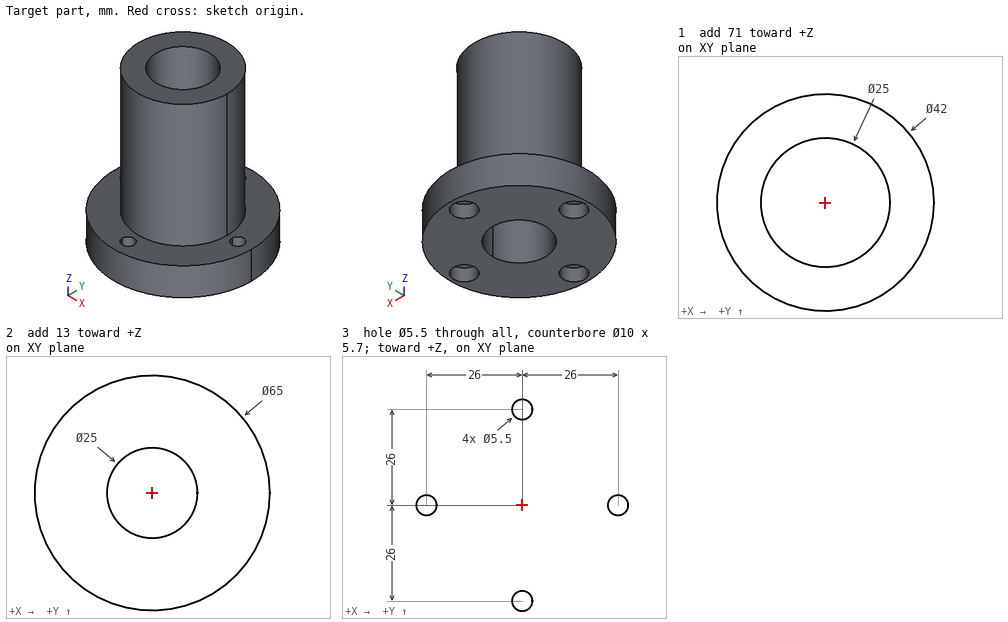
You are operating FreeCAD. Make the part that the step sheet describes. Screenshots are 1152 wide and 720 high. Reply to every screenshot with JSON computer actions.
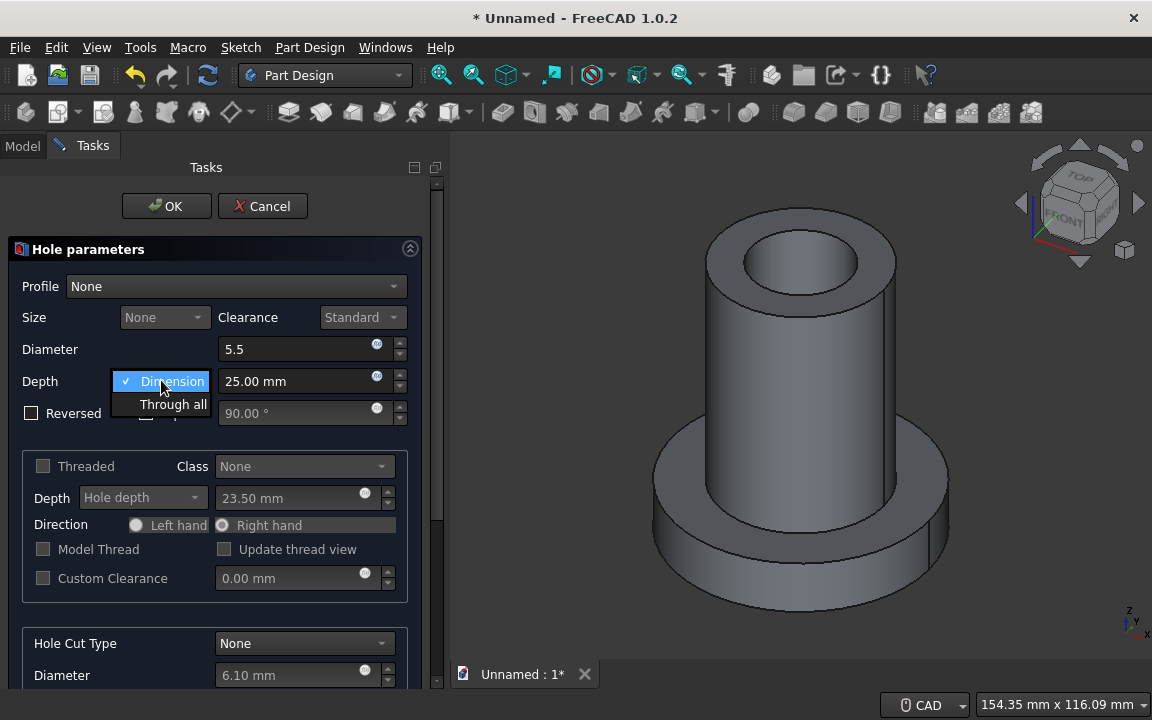
{"action": "left_click", "coordinate": [160, 404]}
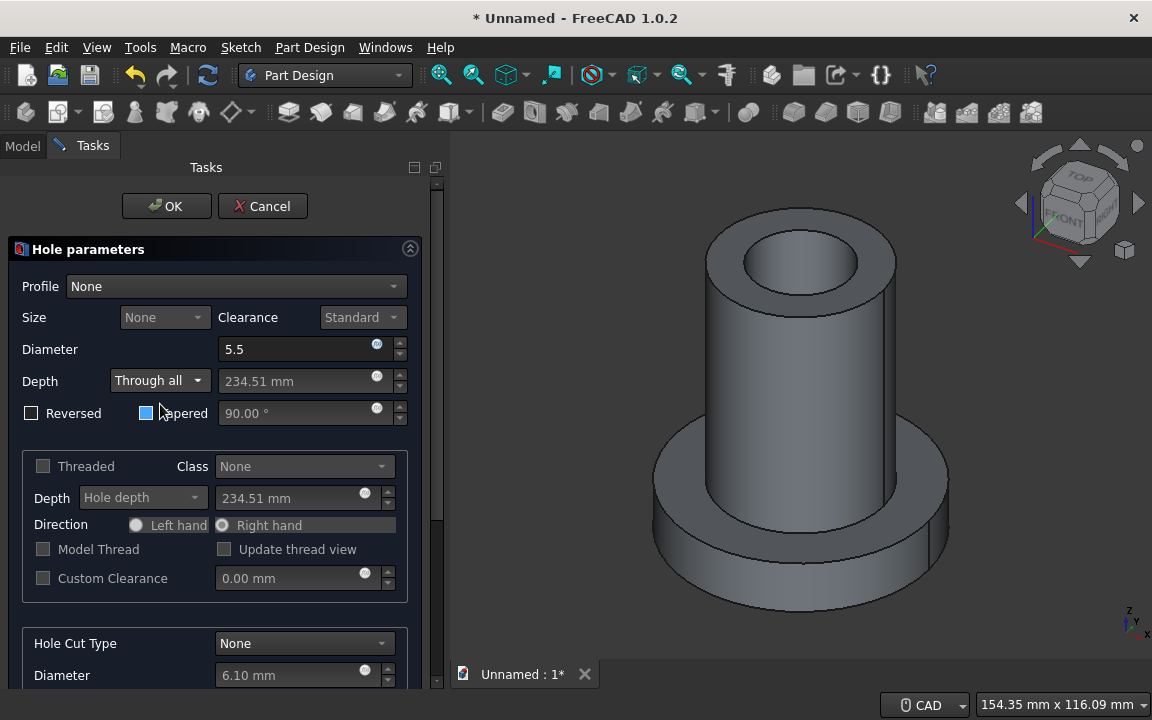
{"action": "left_click", "coordinate": [30, 413]}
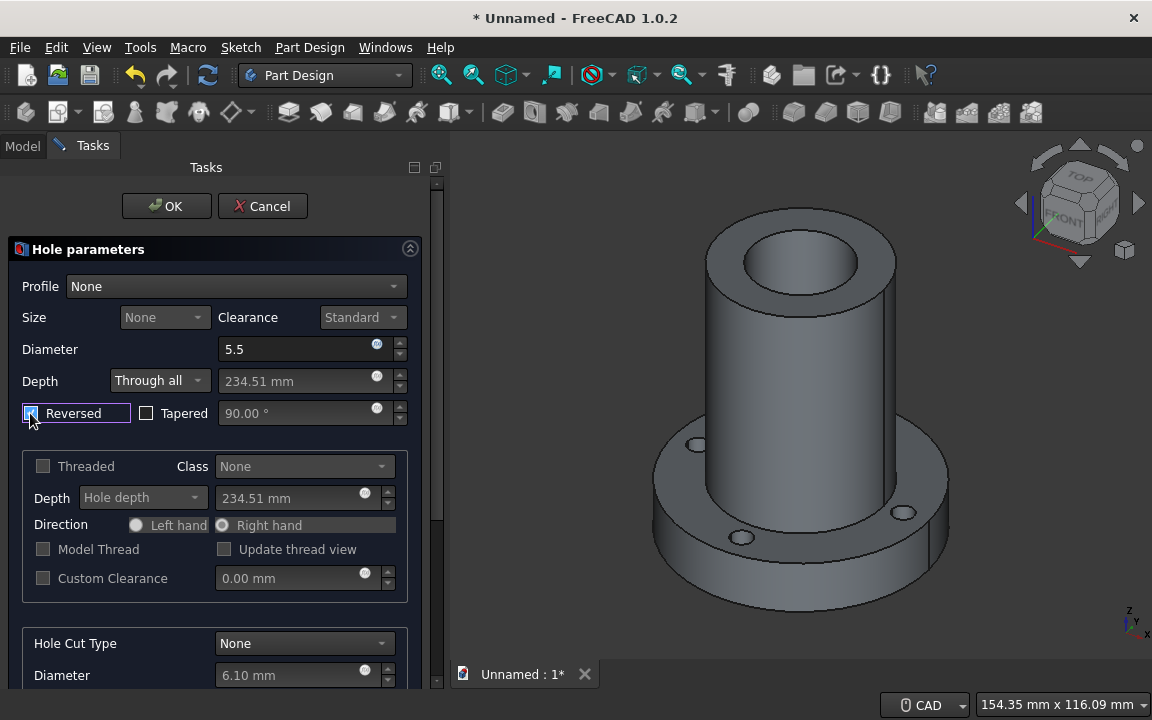
{"action": "left_click", "coordinate": [306, 644]}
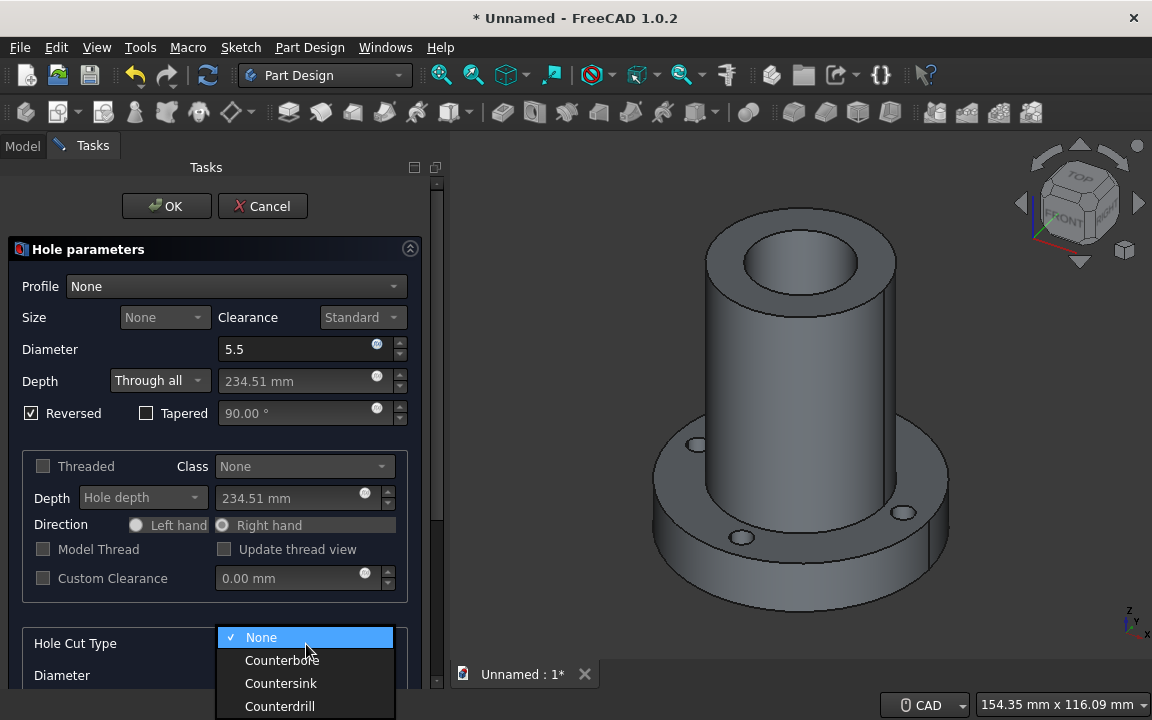
{"action": "left_click", "coordinate": [304, 660]}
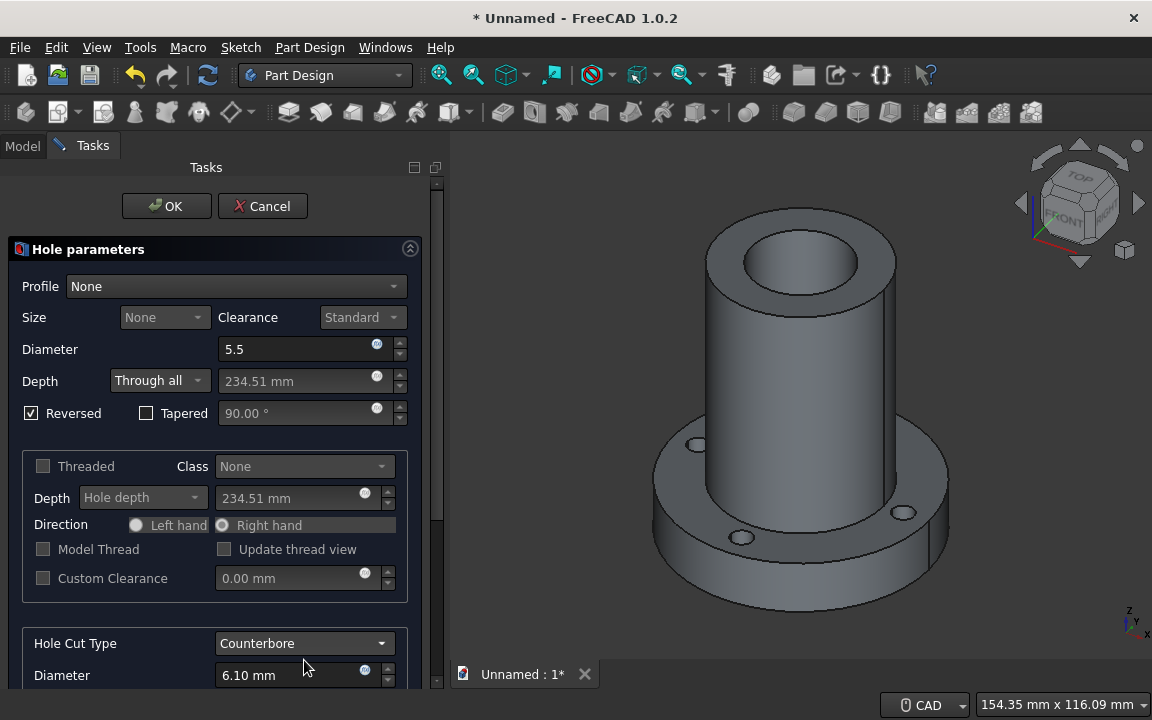
{"action": "triple_click", "coordinate": [298, 675]}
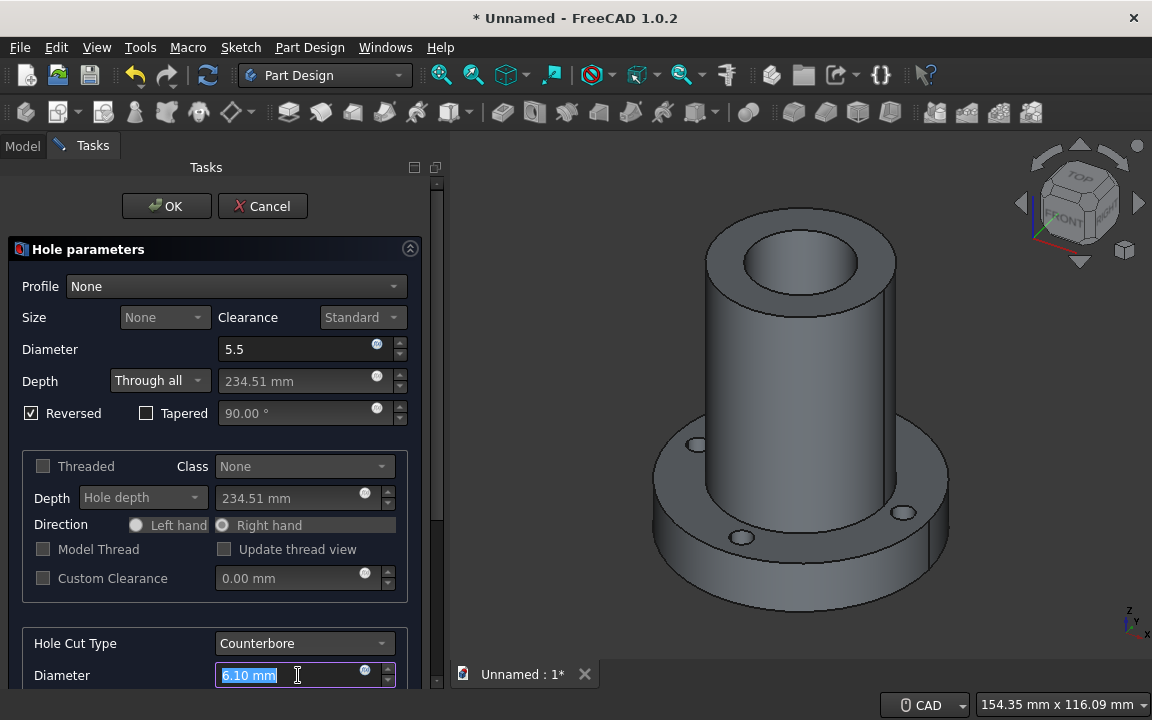
{"action": "type", "text": "10"}
{"action": "key", "text": "Tab"}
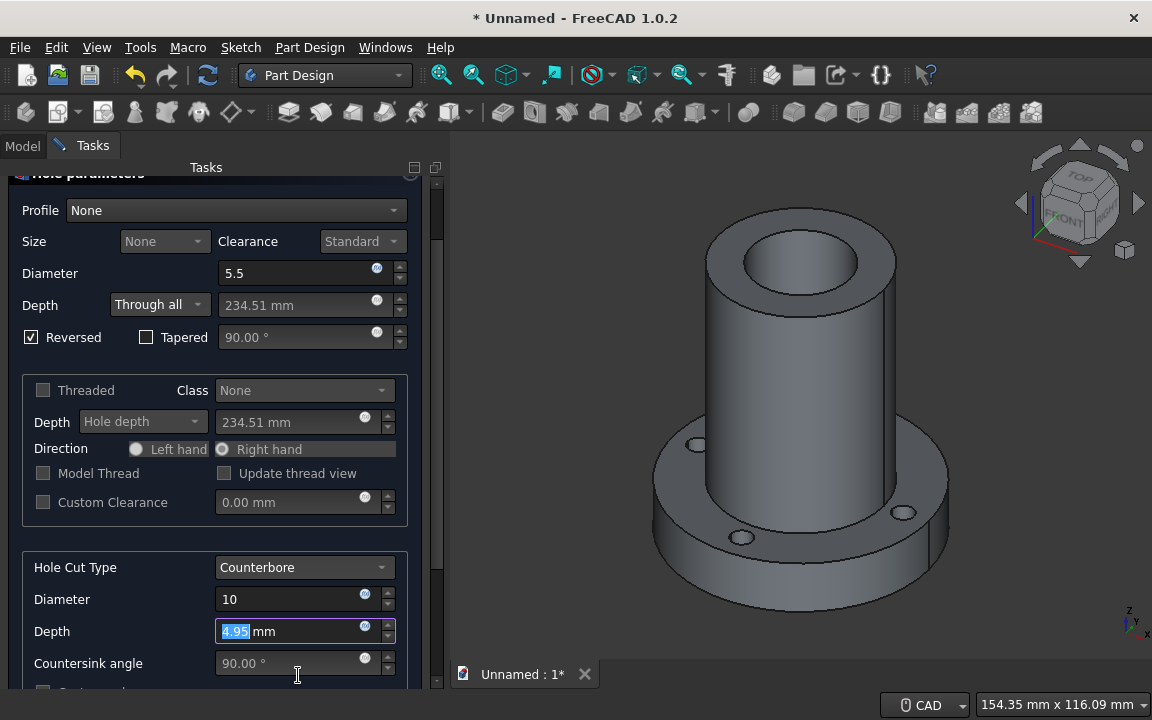
{"action": "type", "text": "5.7"}
{"action": "key", "text": "Tab"}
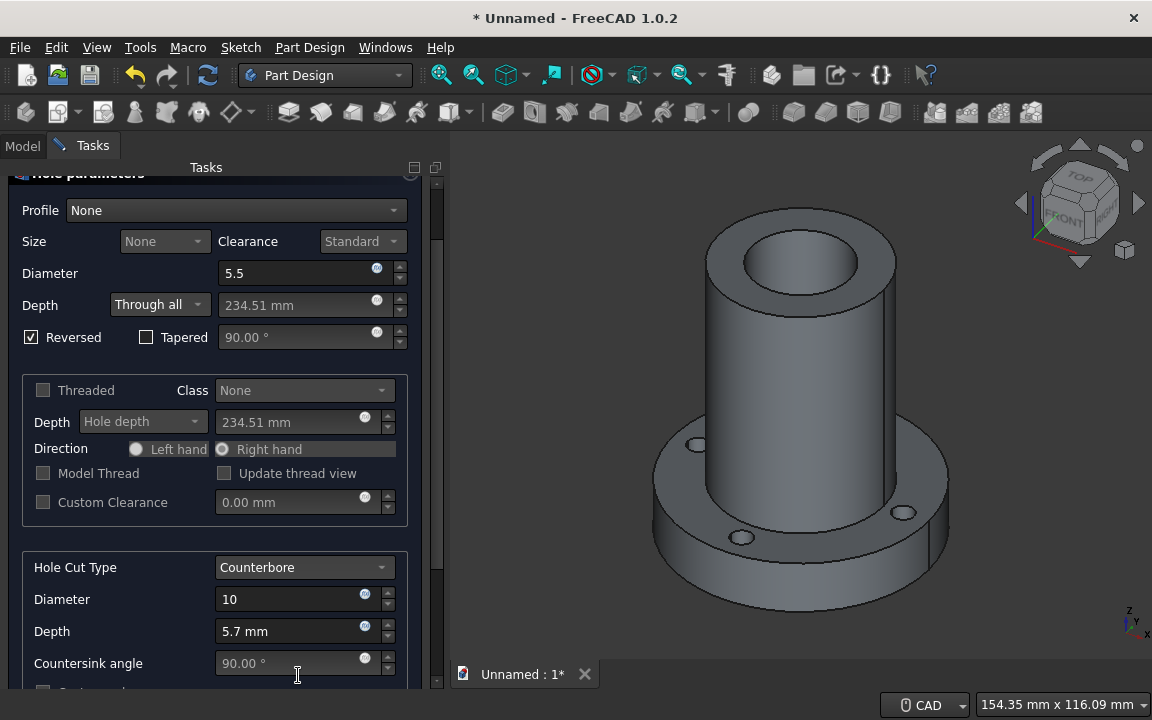
{"action": "scroll", "coordinate": [437, 432], "scroll_direction": "up", "scroll_amount": 3}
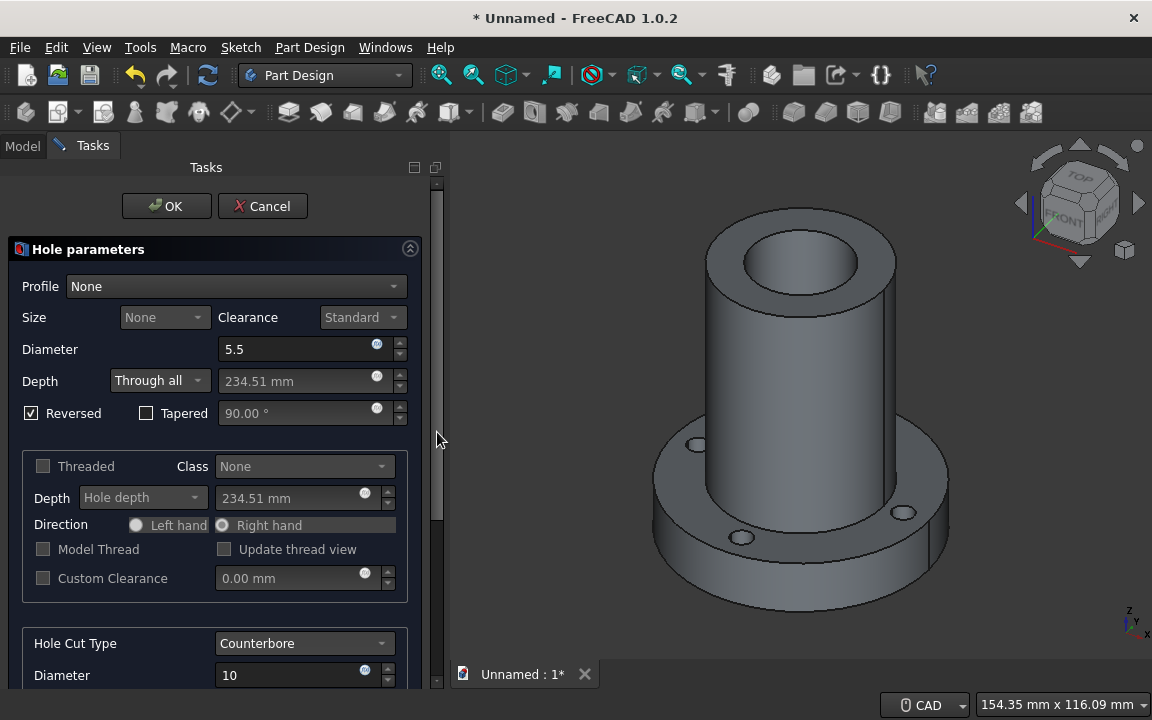
{"action": "left_click", "coordinate": [167, 206]}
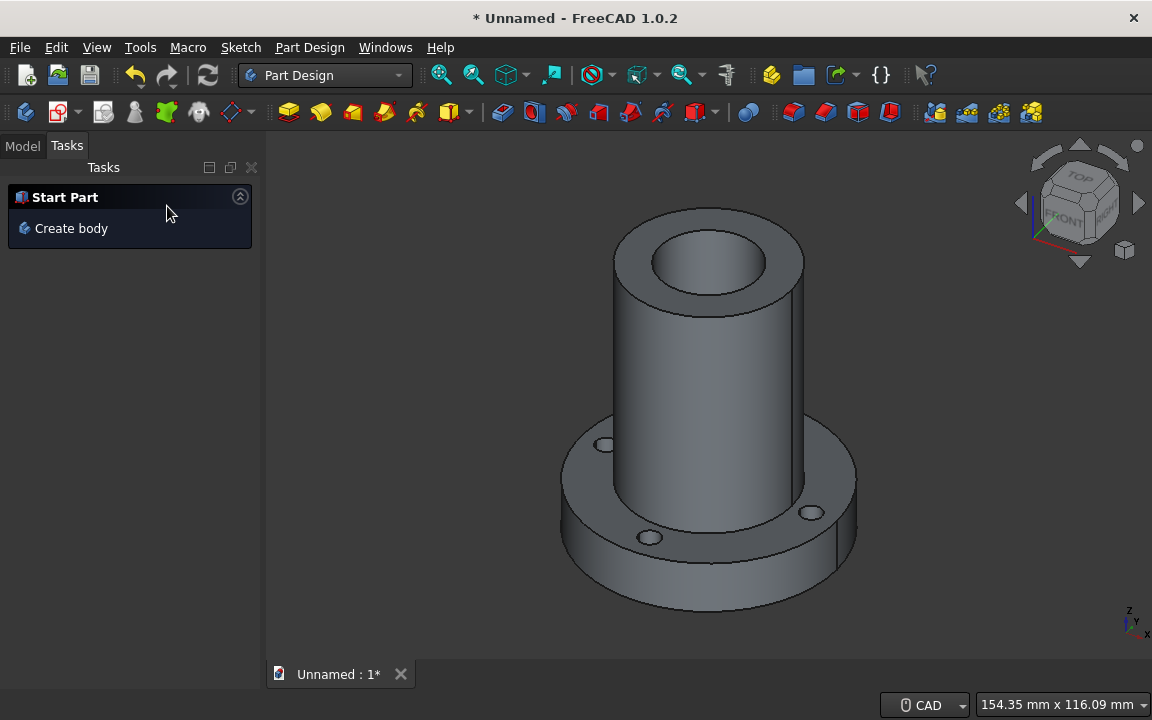
{"action": "key", "text": "0"}